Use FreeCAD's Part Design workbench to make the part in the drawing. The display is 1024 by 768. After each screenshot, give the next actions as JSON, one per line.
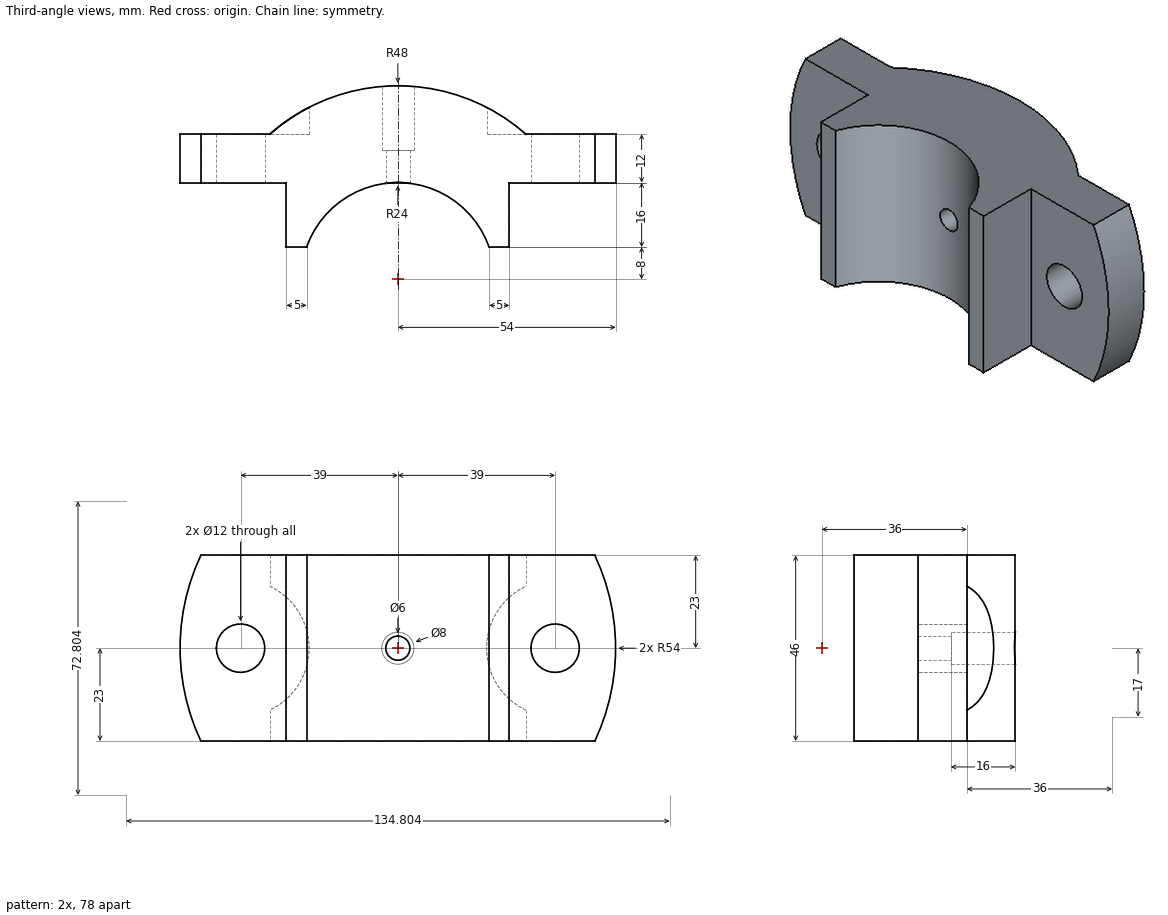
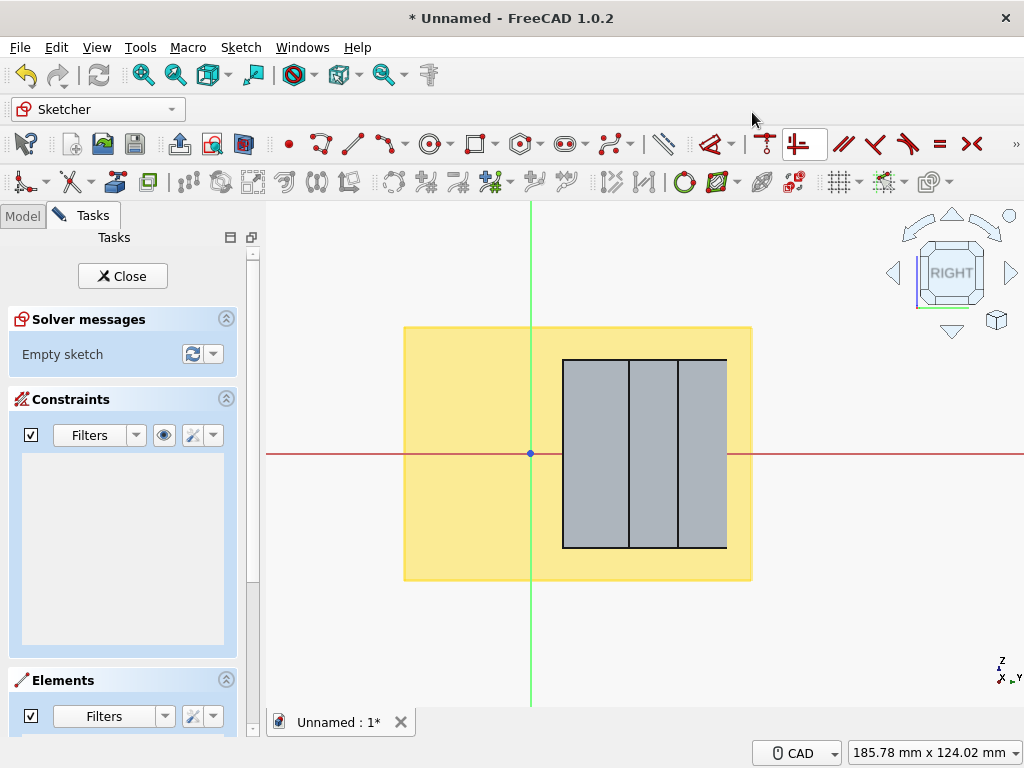
{"action": "left_click", "coordinate": [244, 144]}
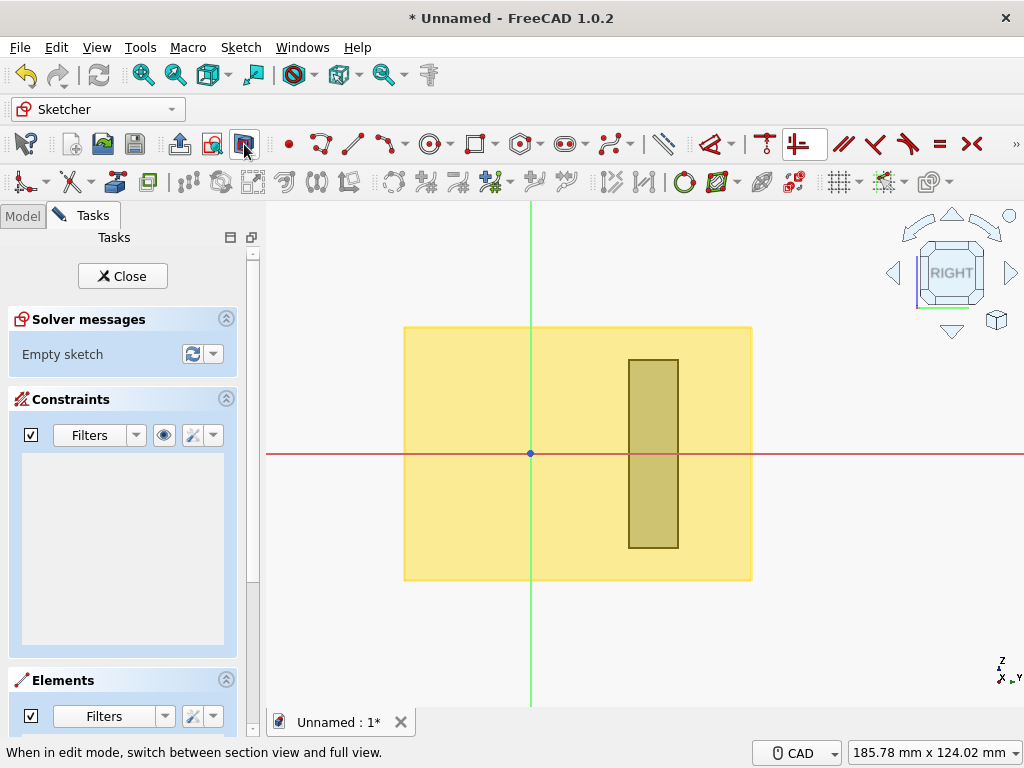
{"action": "scroll", "coordinate": [859, 559], "scroll_direction": "up", "scroll_amount": 2}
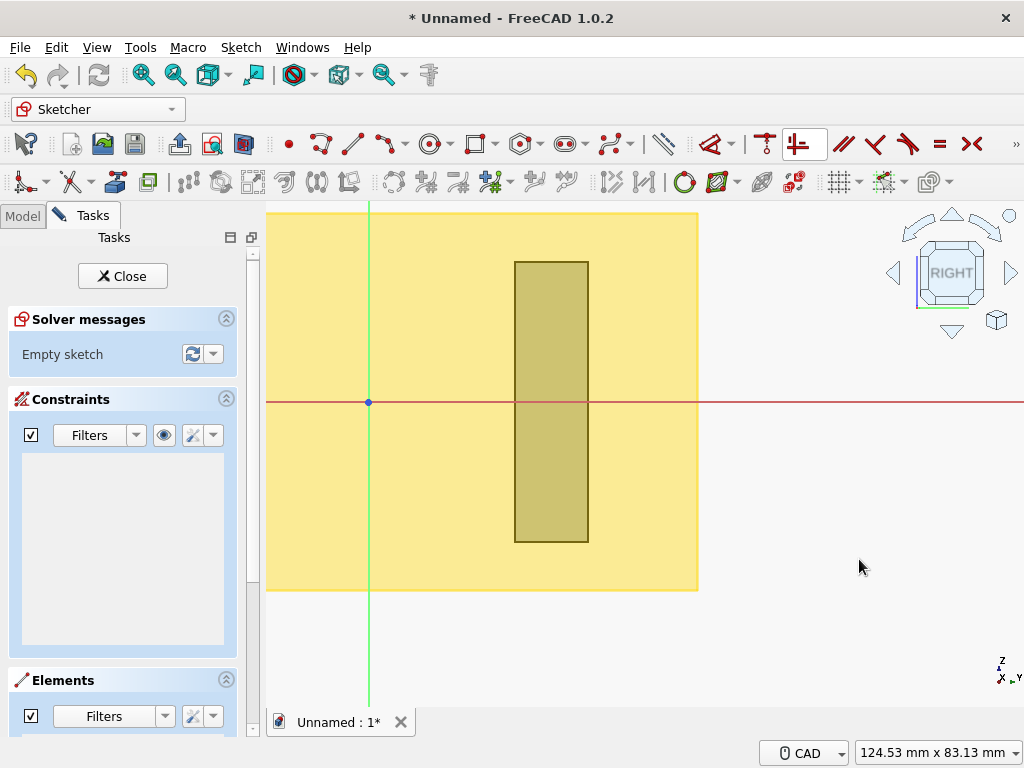
{"action": "left_click", "coordinate": [476, 144]}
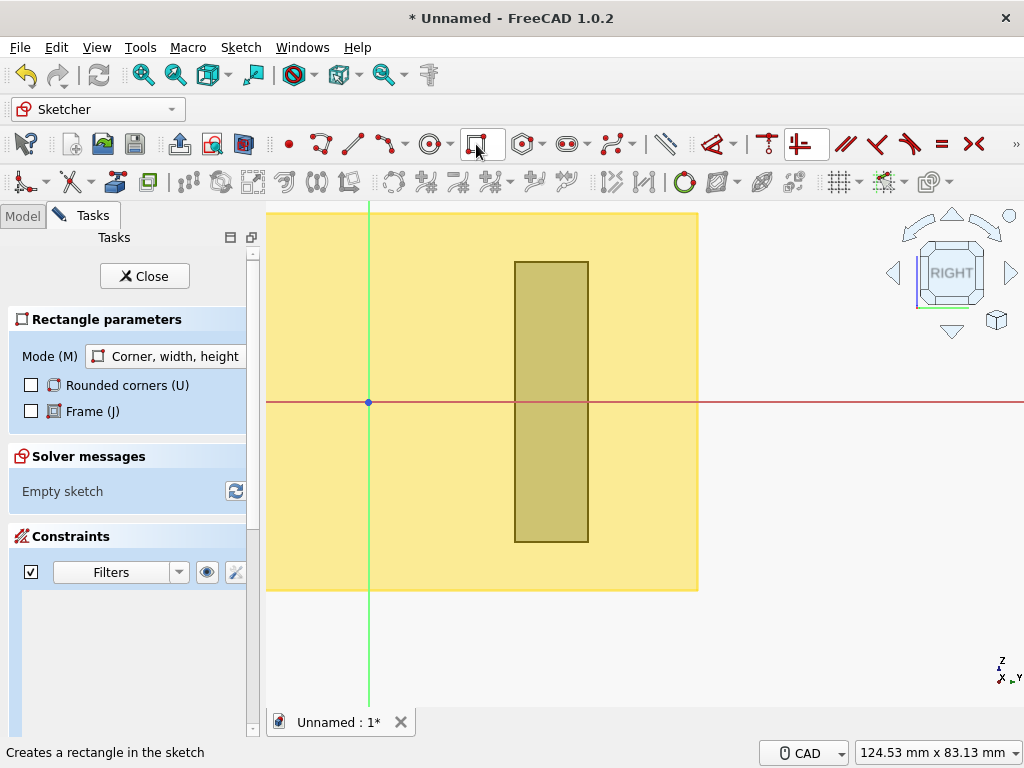
{"action": "left_click", "coordinate": [588, 402]}
{"action": "mouse_move", "coordinate": [807, 505]}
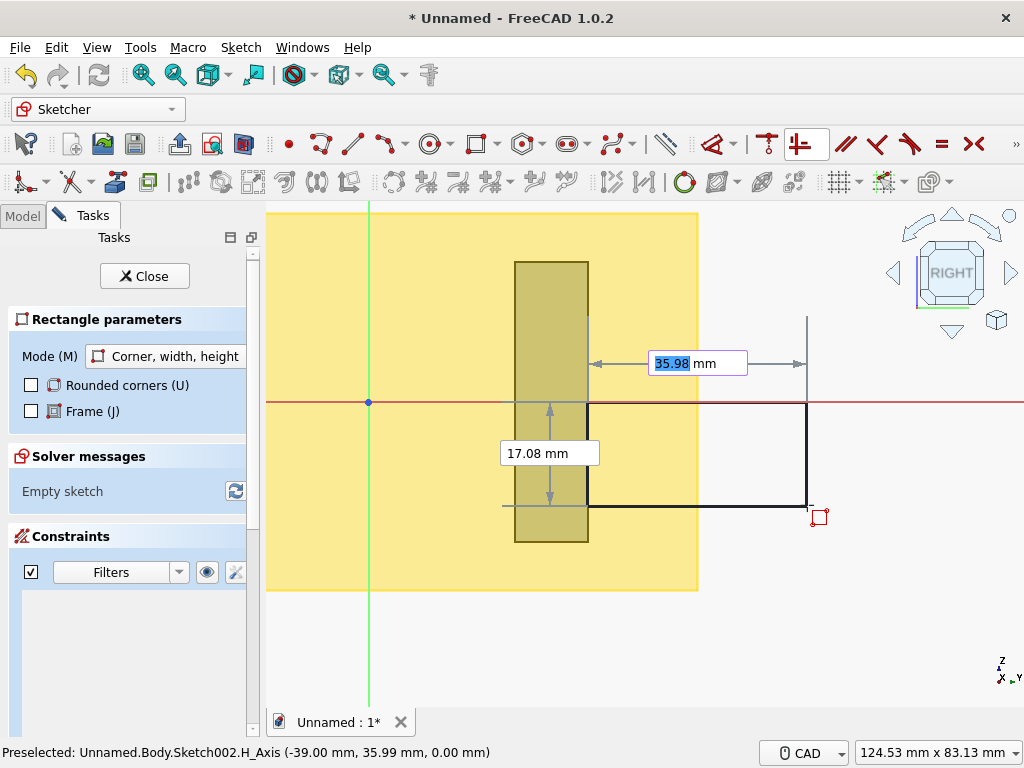
{"action": "type", "text": "36"}
{"action": "key", "text": "Tab"}
{"action": "type", "text": "17"}
{"action": "key", "text": "Return"}
{"action": "key", "text": "Escape"}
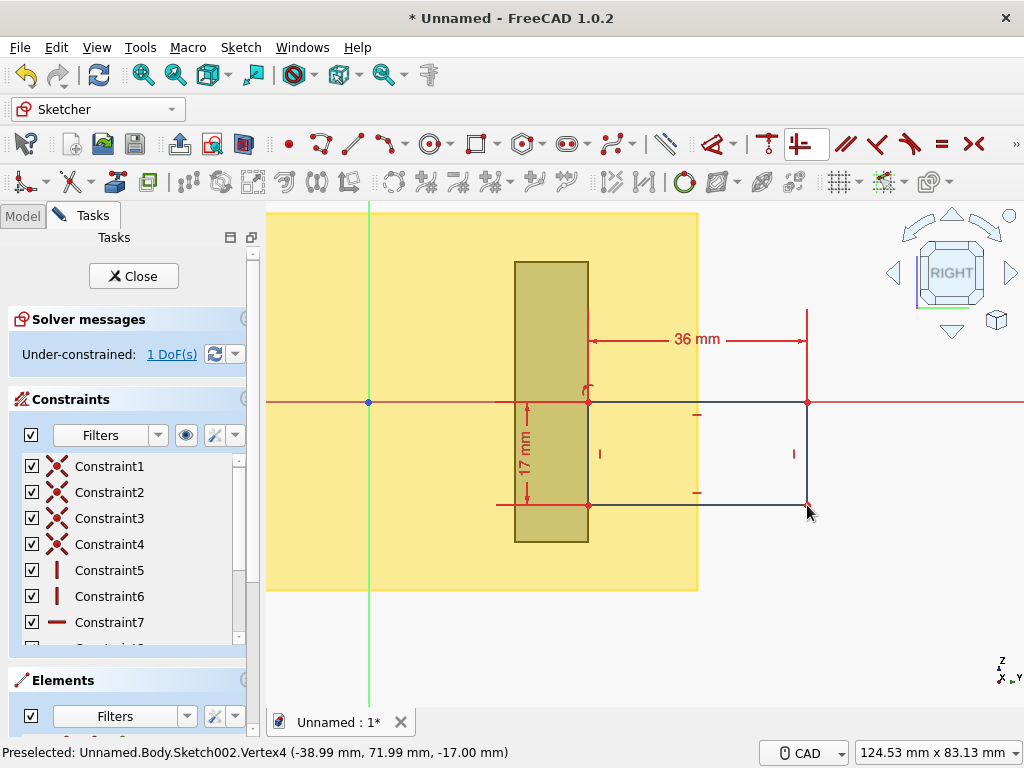
{"action": "key", "text": "d"}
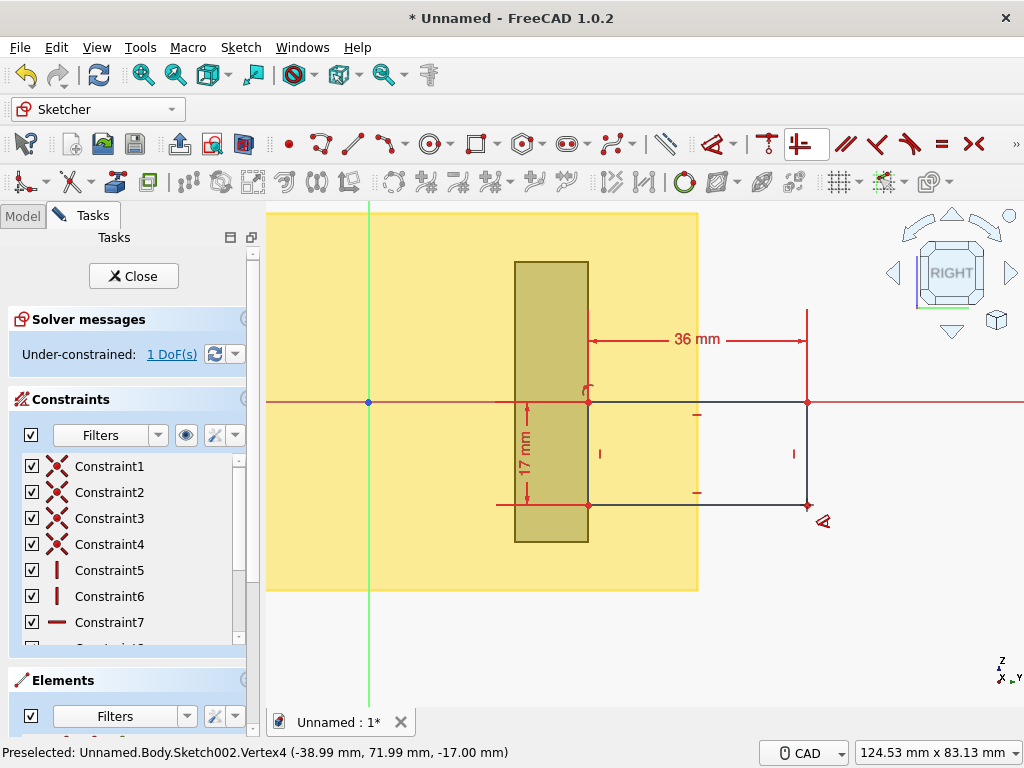
{"action": "left_click", "coordinate": [588, 402]}
{"action": "left_click", "coordinate": [478, 368]}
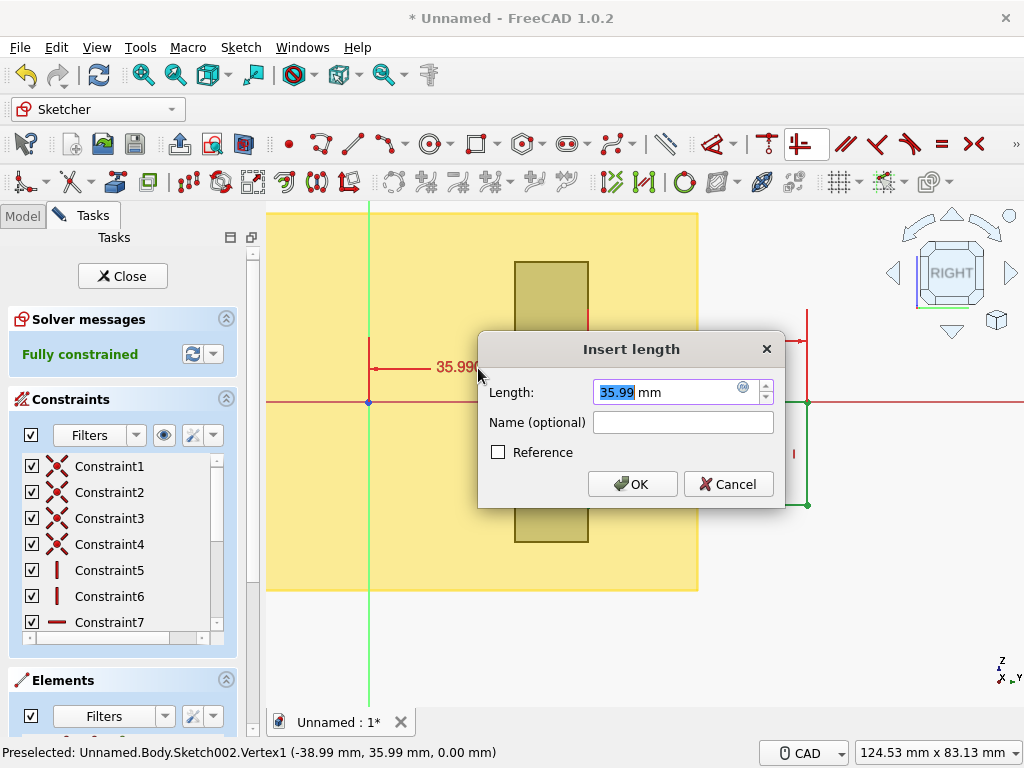
{"action": "type", "text": "36"}
{"action": "key", "text": "Return"}
{"action": "key", "text": "Escape"}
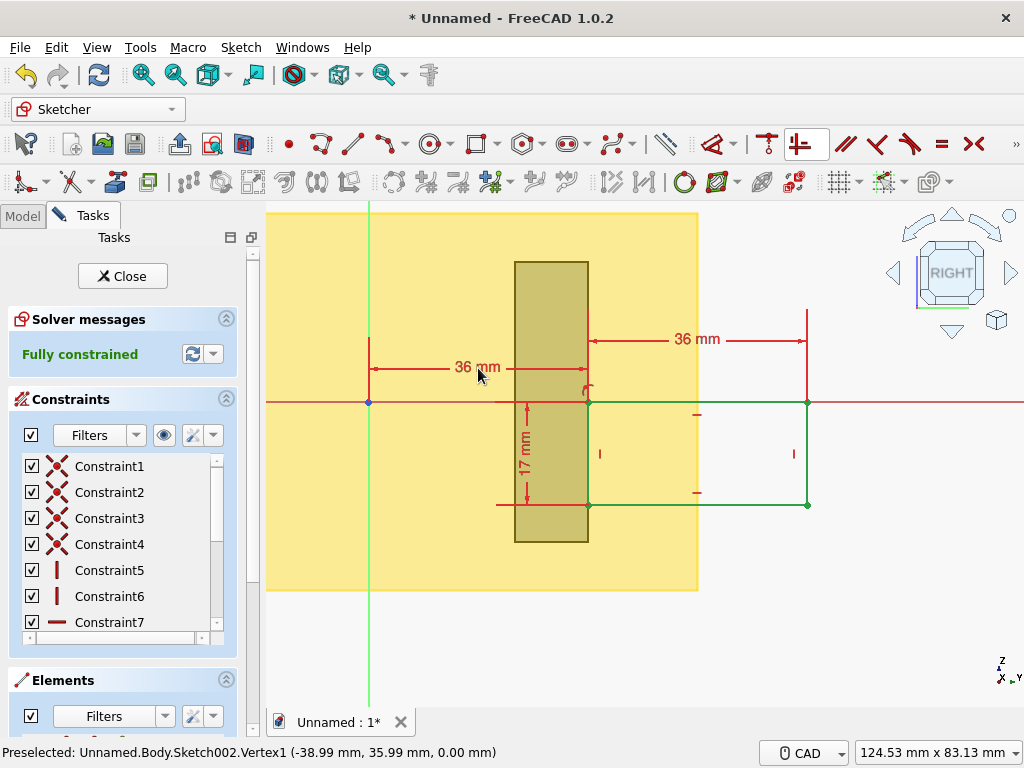
{"action": "left_click", "coordinate": [123, 276]}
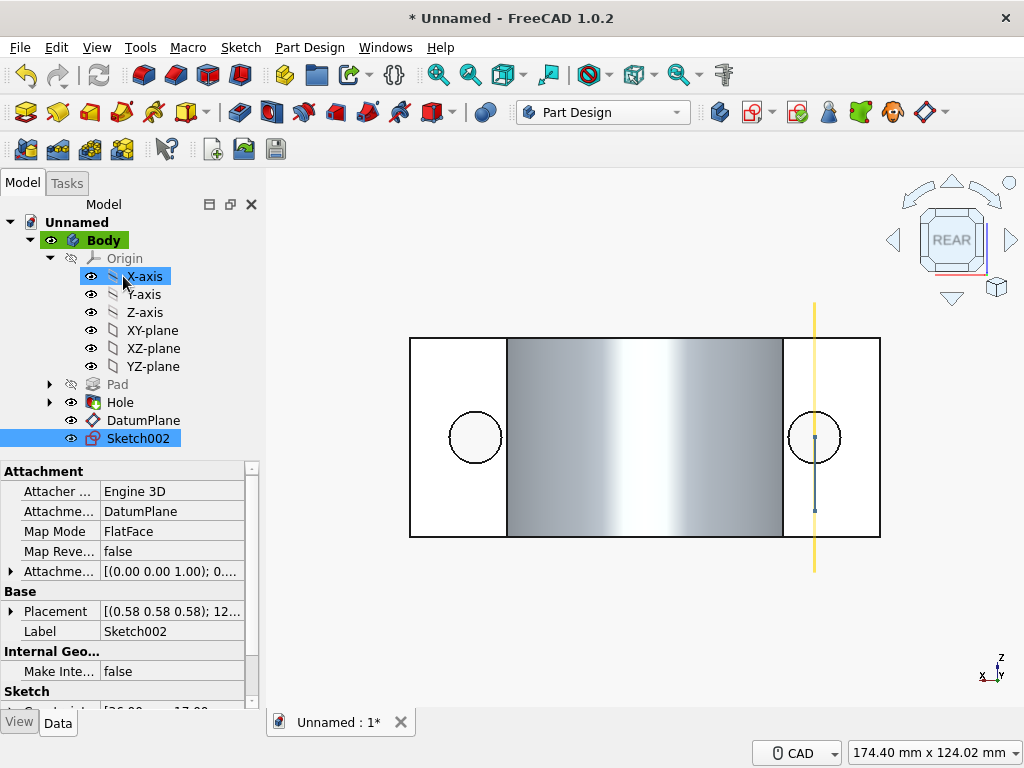
{"action": "left_click", "coordinate": [304, 112]}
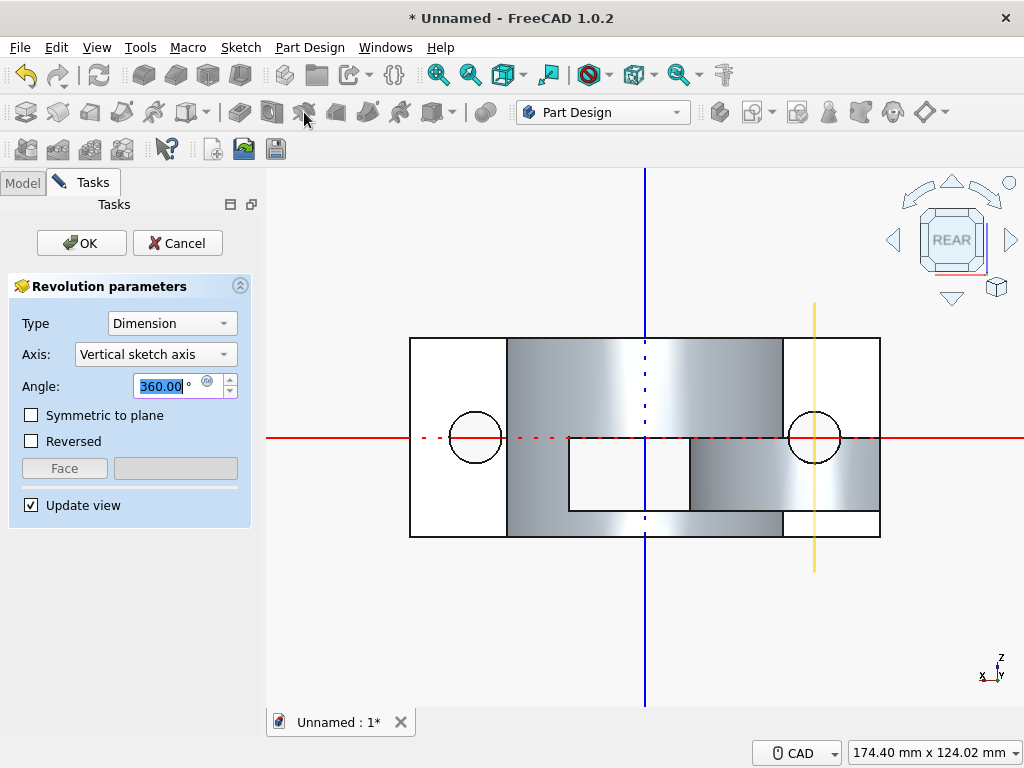
{"action": "left_click", "coordinate": [156, 354]}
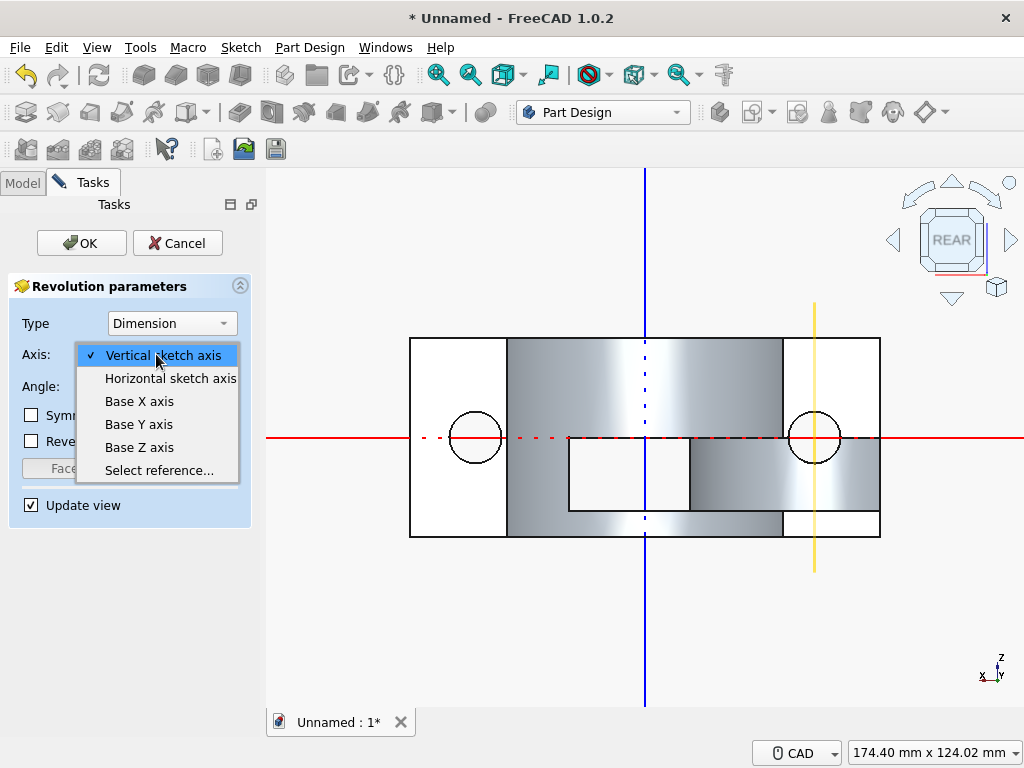
{"action": "left_click", "coordinate": [156, 378]}